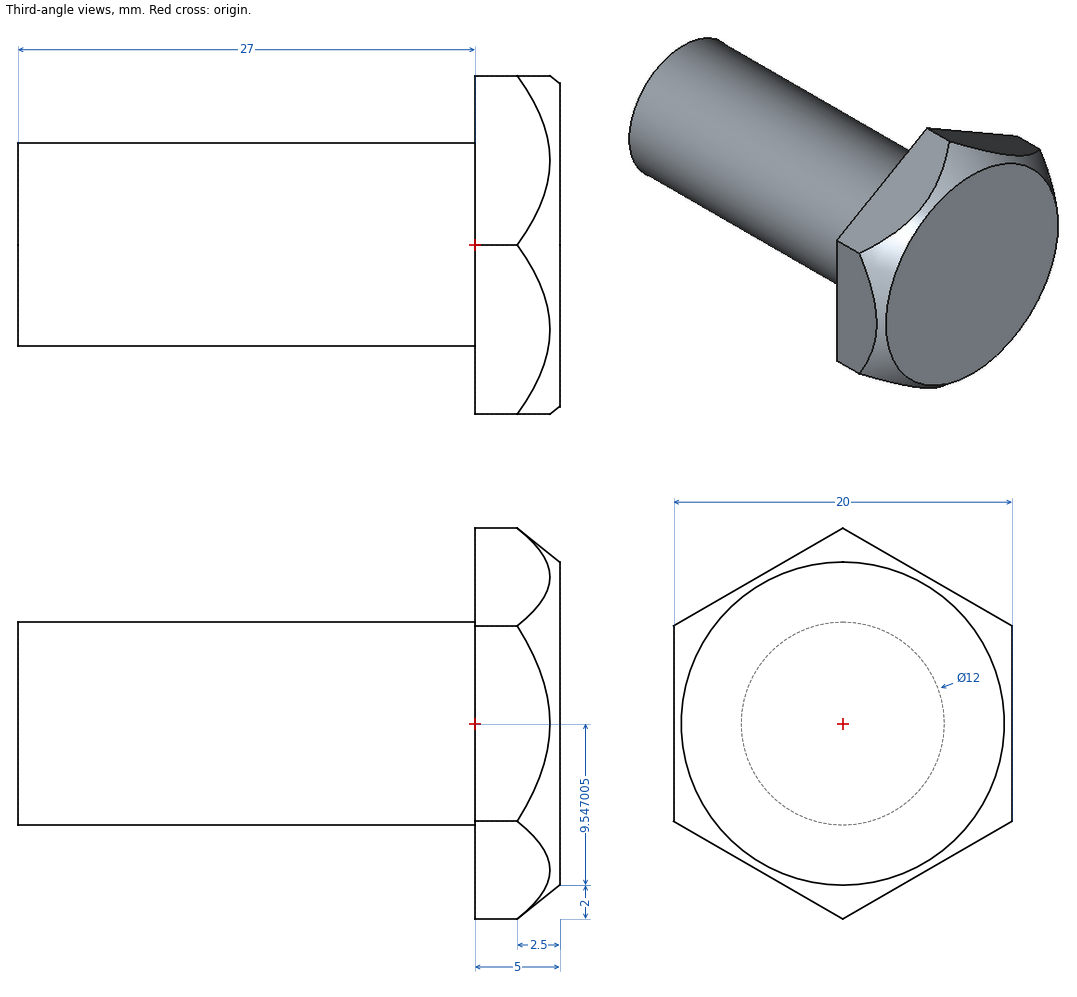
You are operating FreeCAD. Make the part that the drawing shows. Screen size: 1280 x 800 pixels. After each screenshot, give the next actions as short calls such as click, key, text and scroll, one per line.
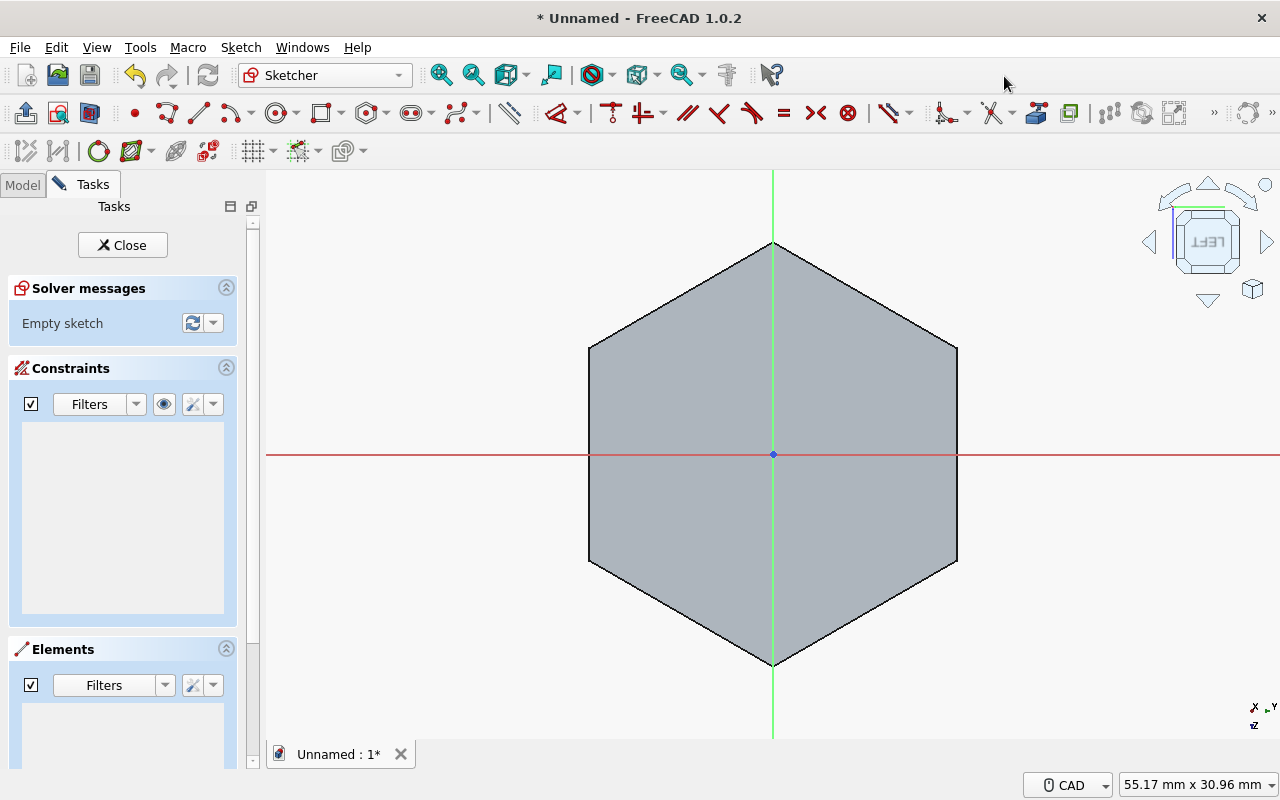
scroll(912, 455, up, 2)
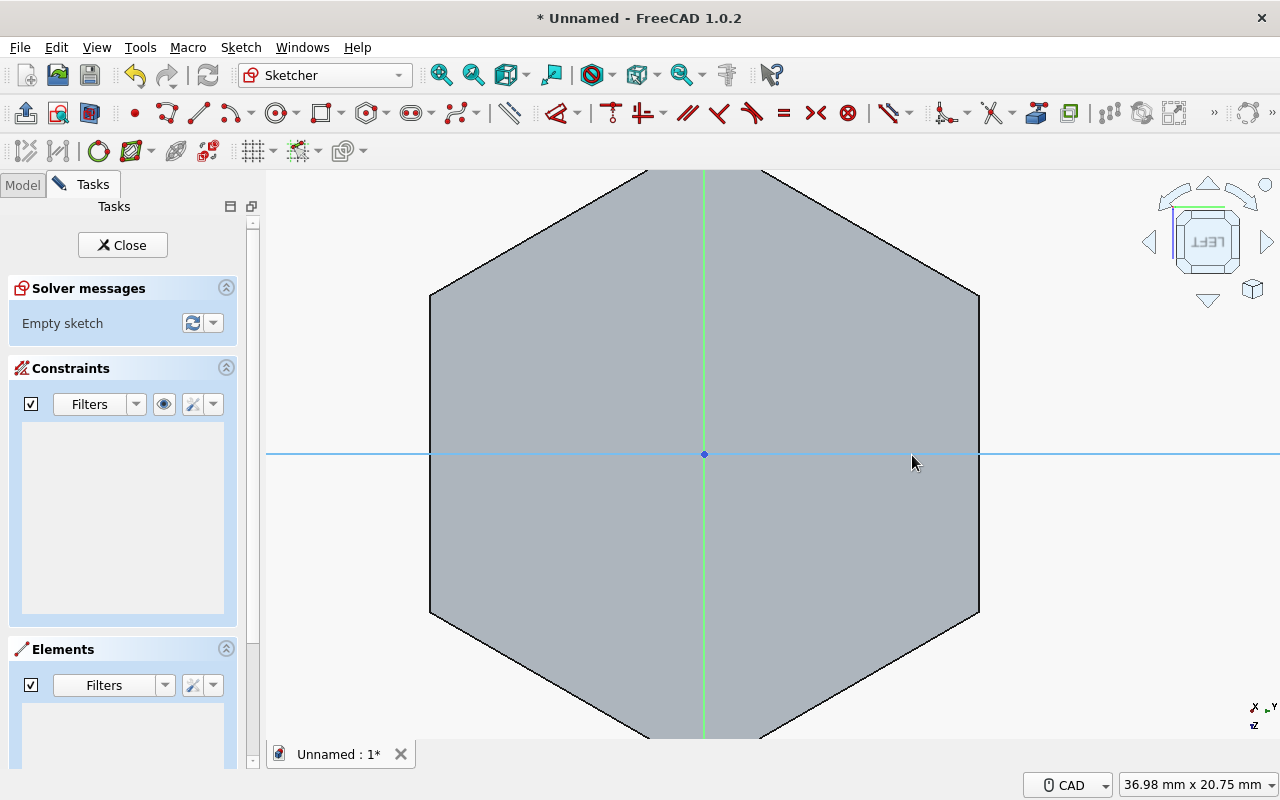
click(276, 114)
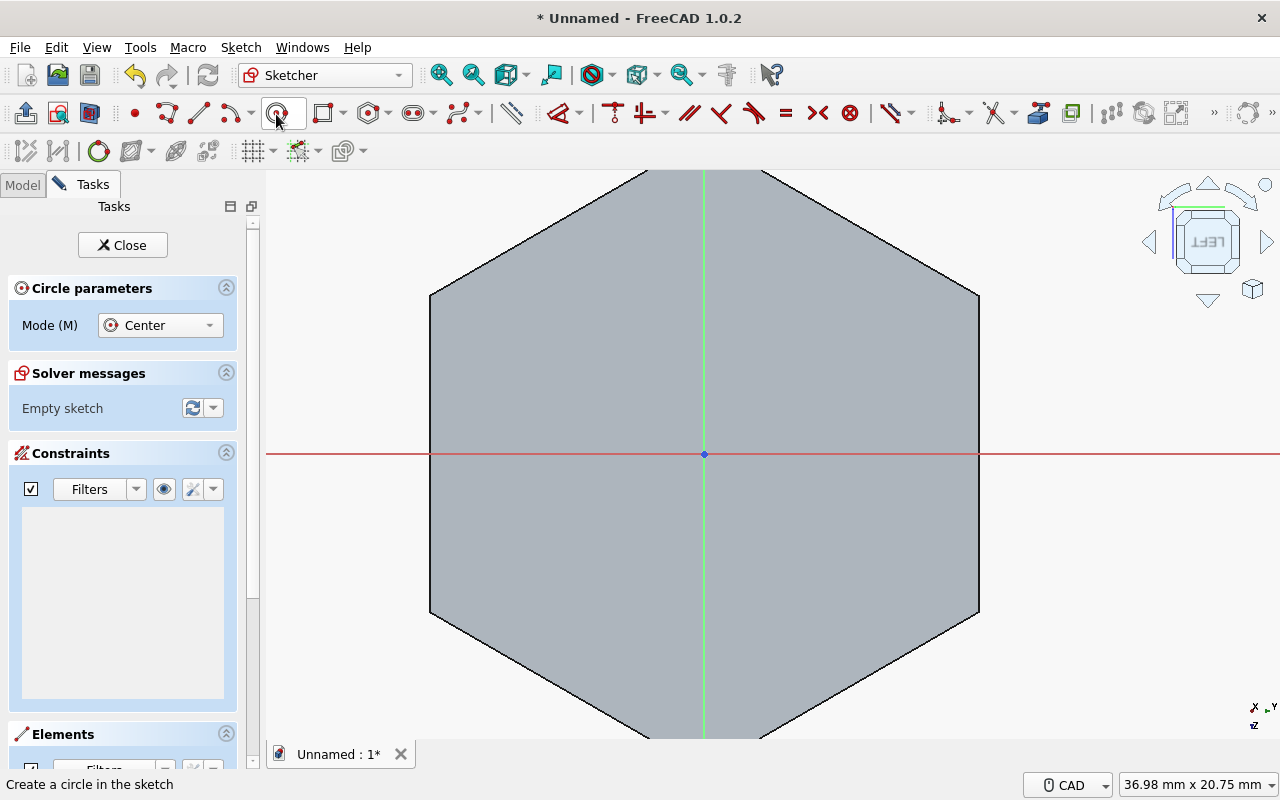
click(704, 454)
click(821, 338)
key(Escape)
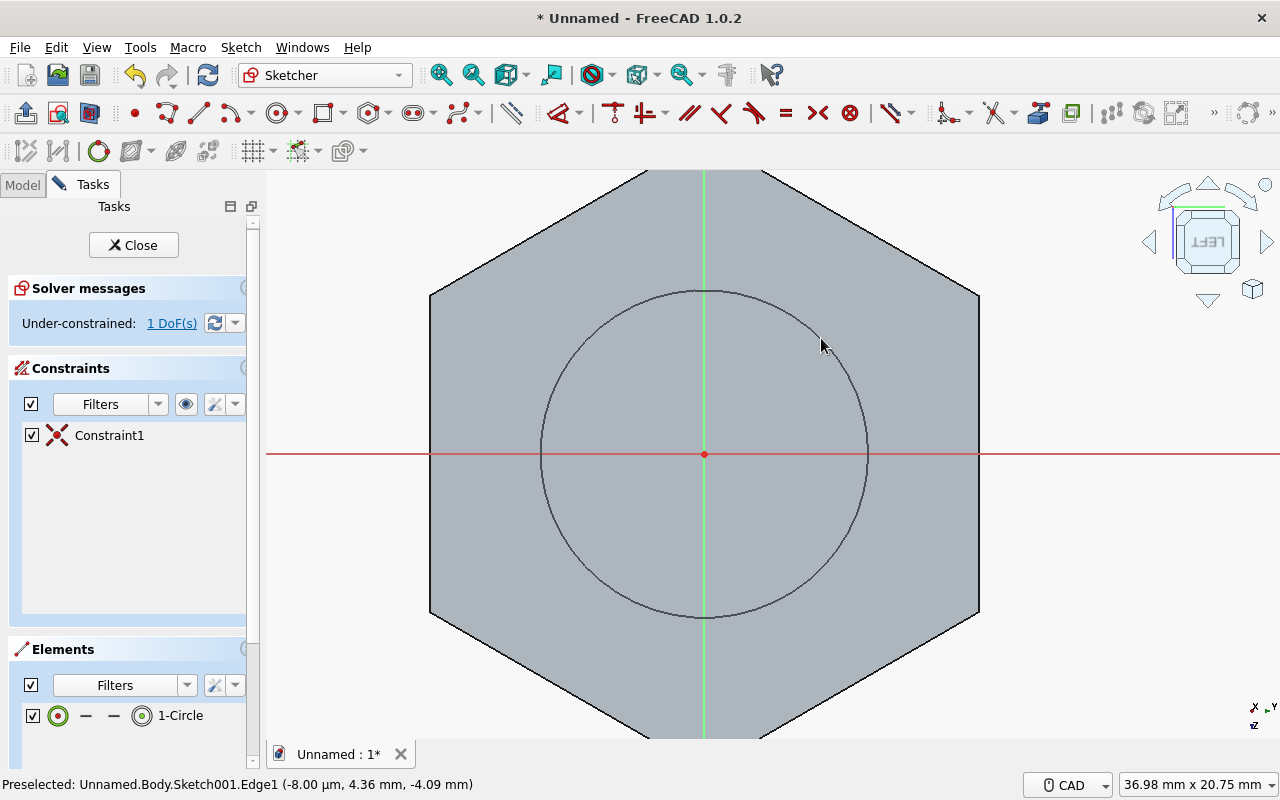
click(558, 114)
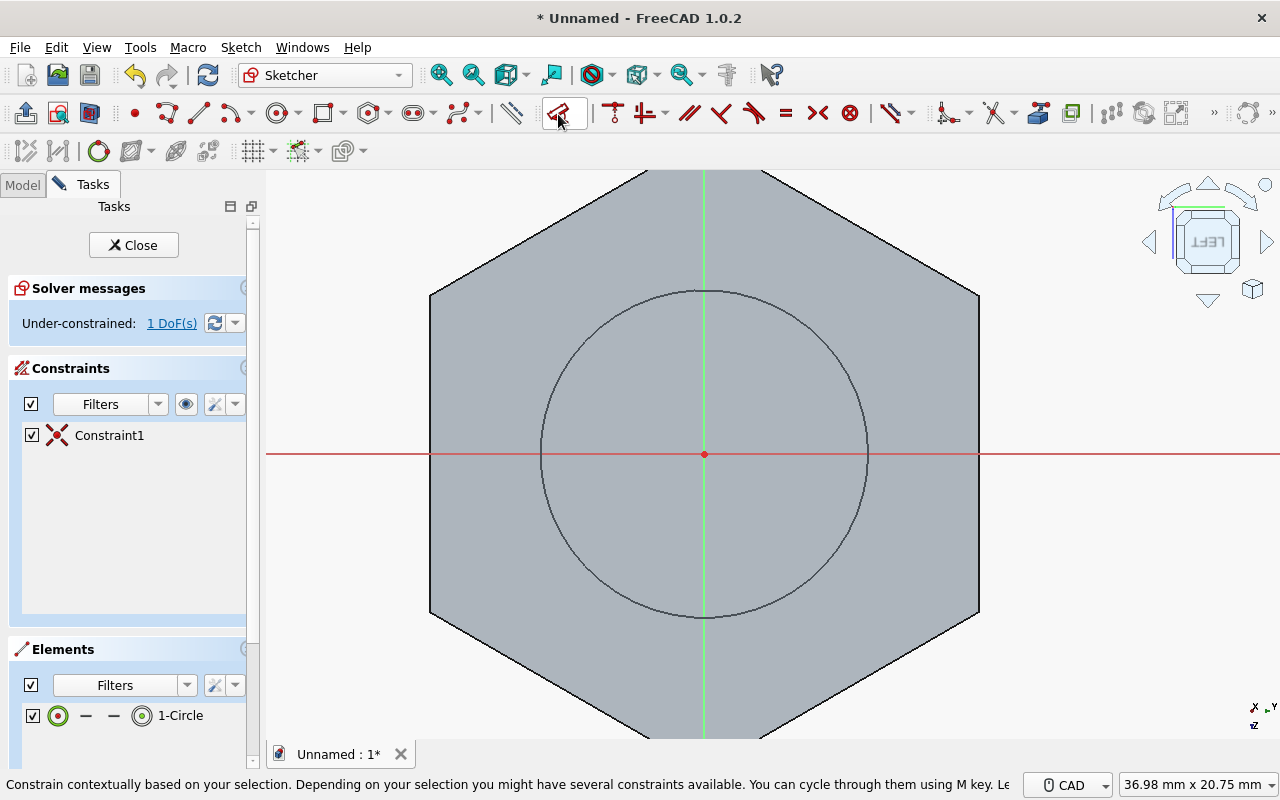
click(820, 338)
click(843, 315)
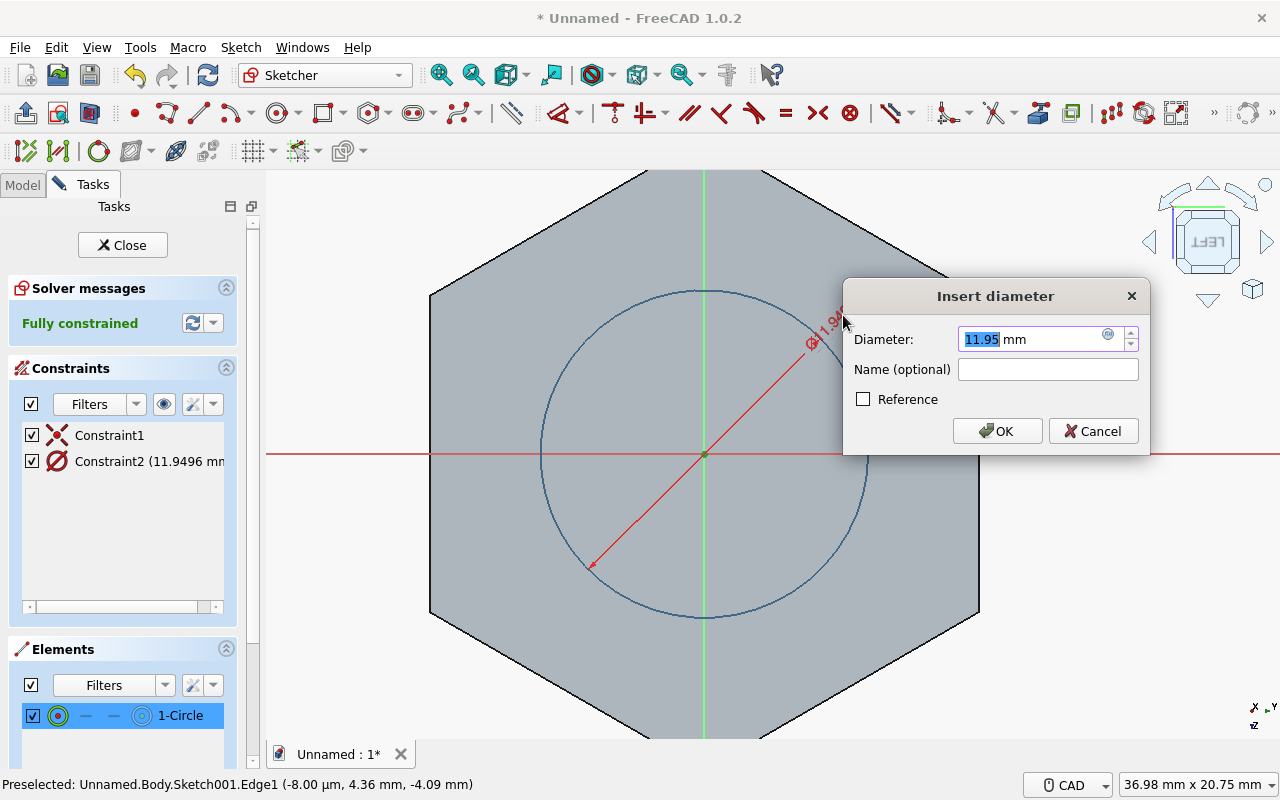
text(12)
key(Return)
key(Escape)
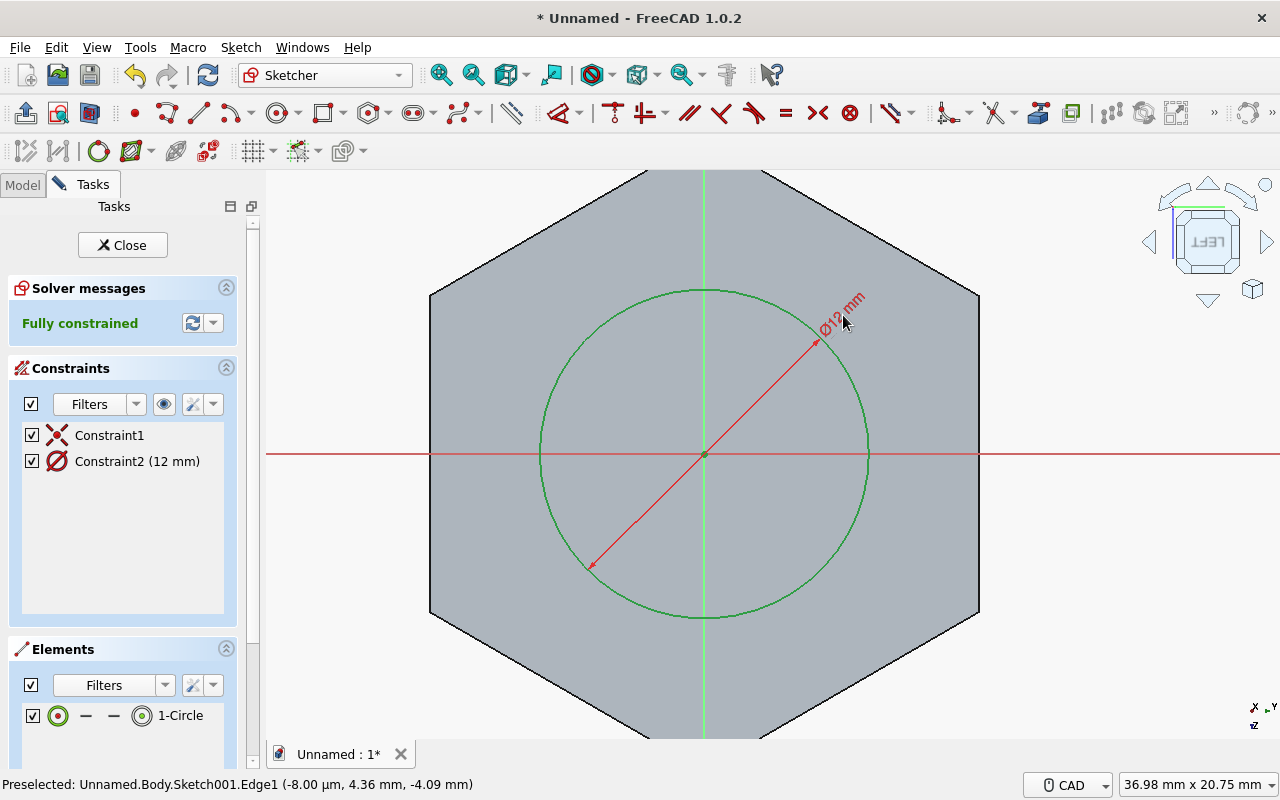
click(123, 245)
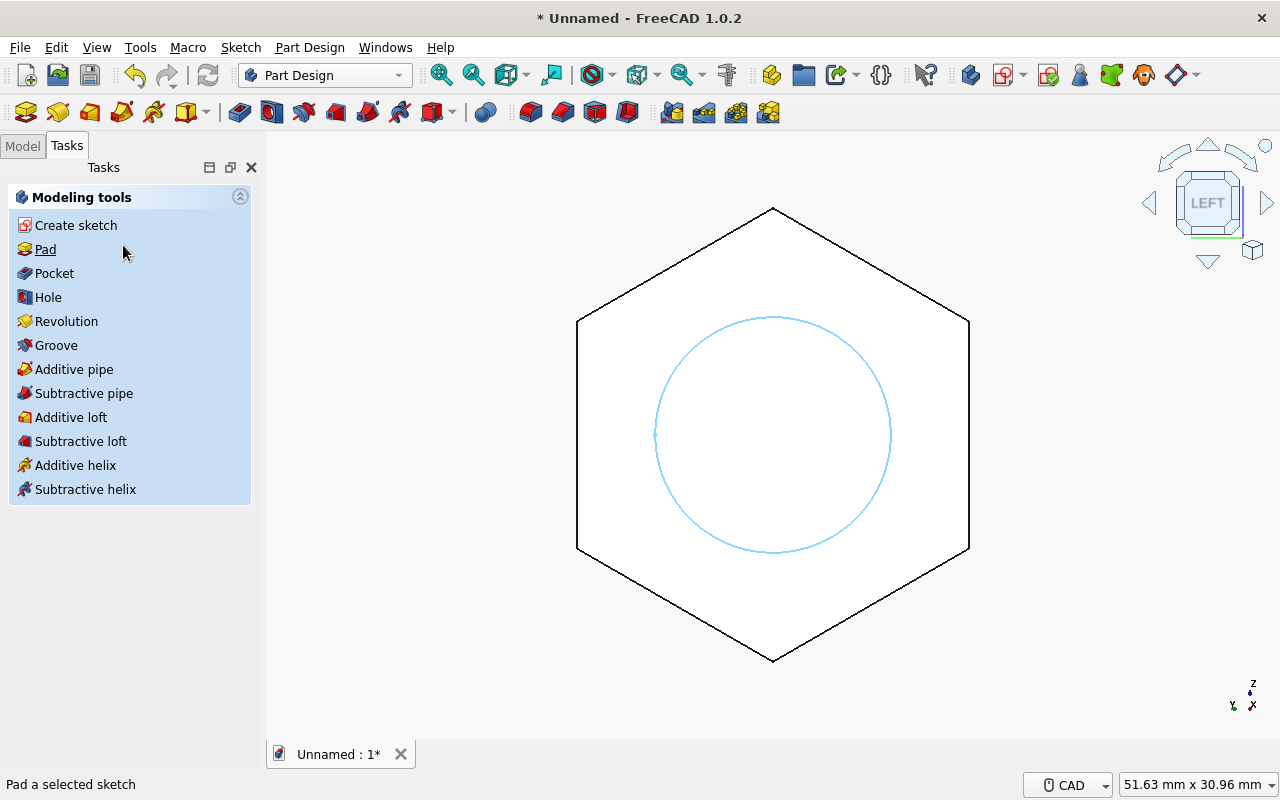
click(26, 112)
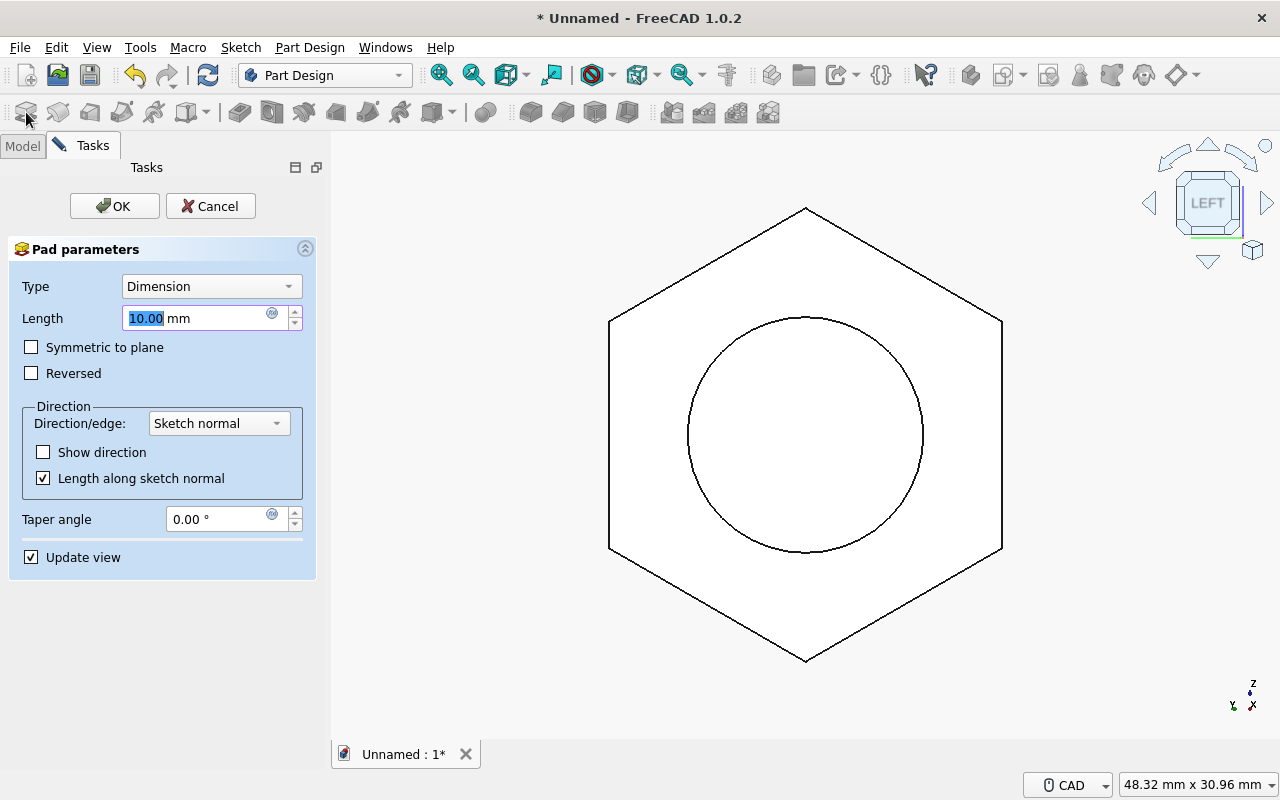
text(27)
key(Tab)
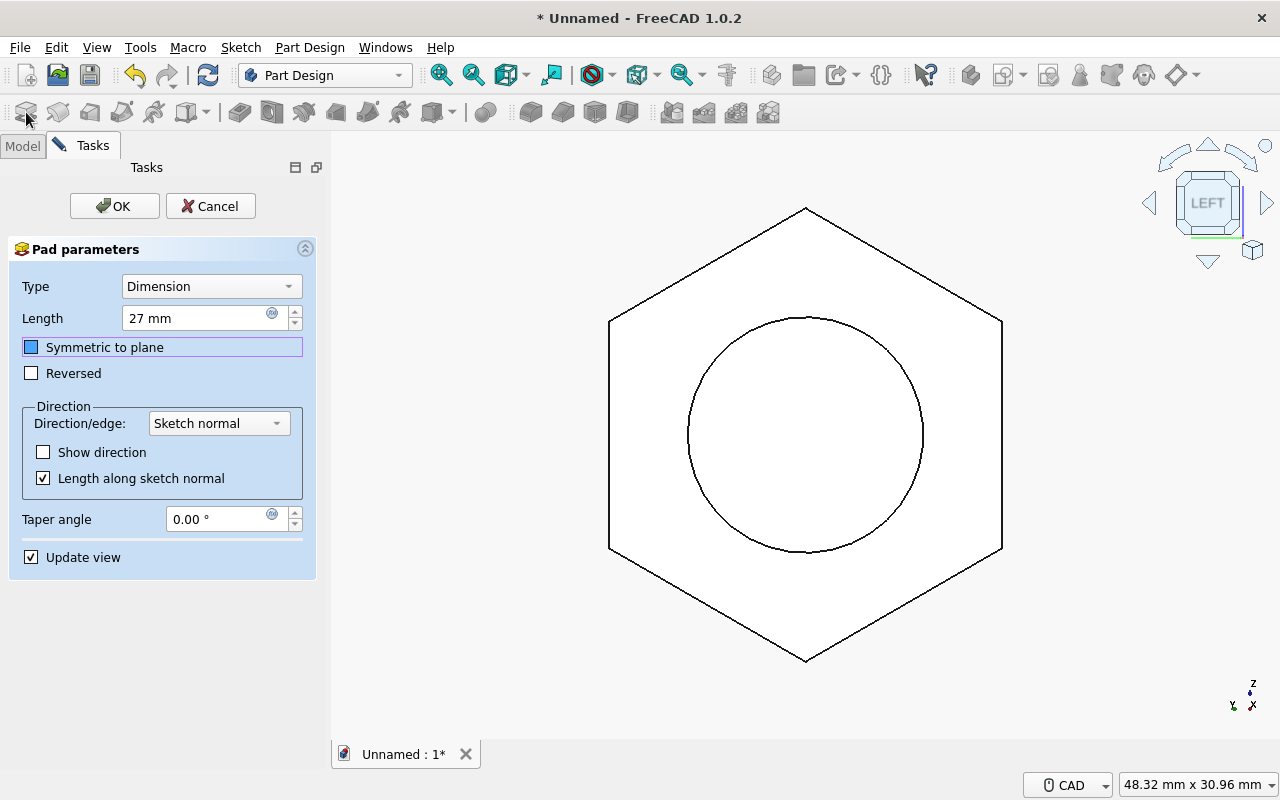
click(115, 206)